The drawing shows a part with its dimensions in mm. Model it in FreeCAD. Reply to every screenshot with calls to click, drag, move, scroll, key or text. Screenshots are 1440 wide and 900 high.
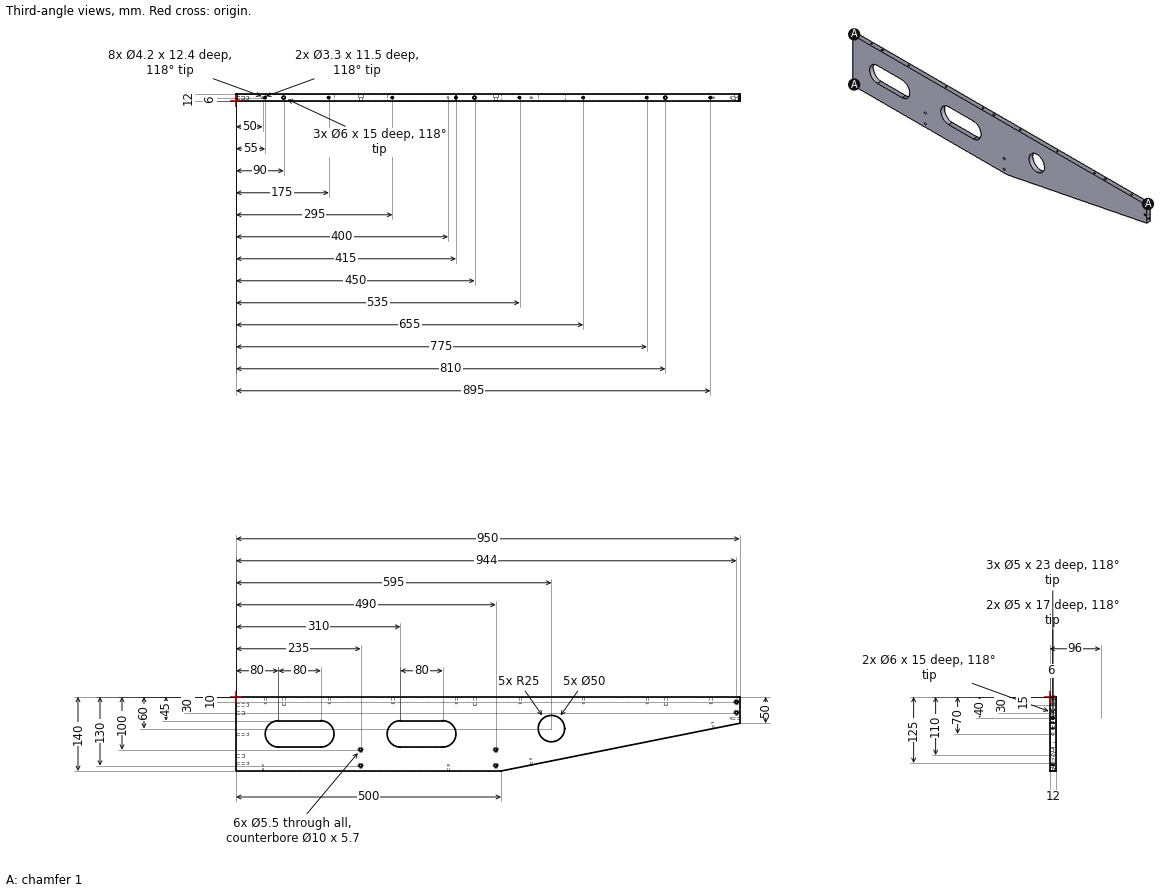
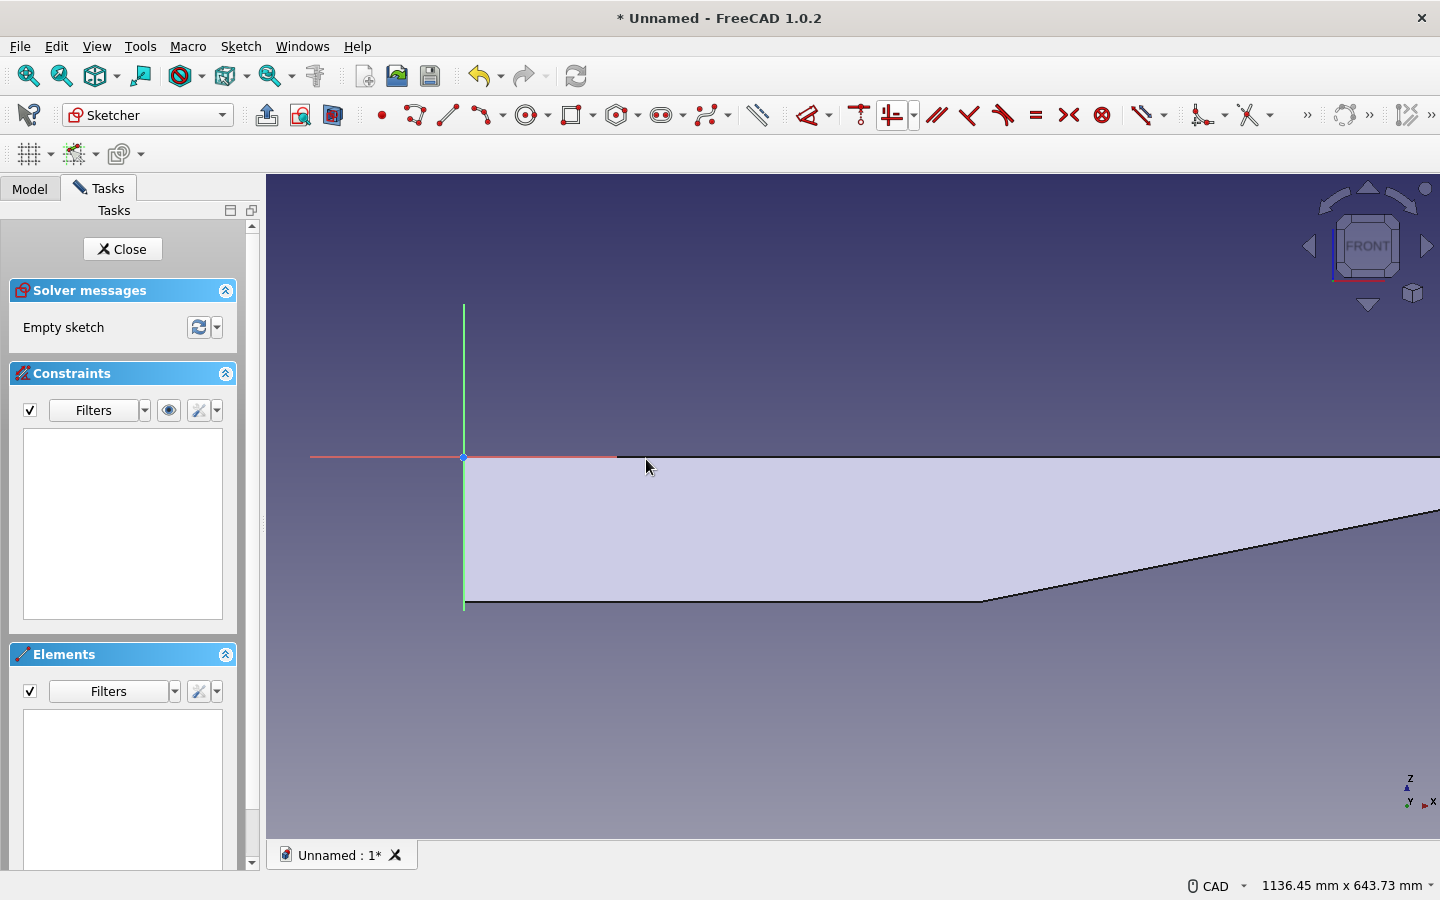
click(660, 116)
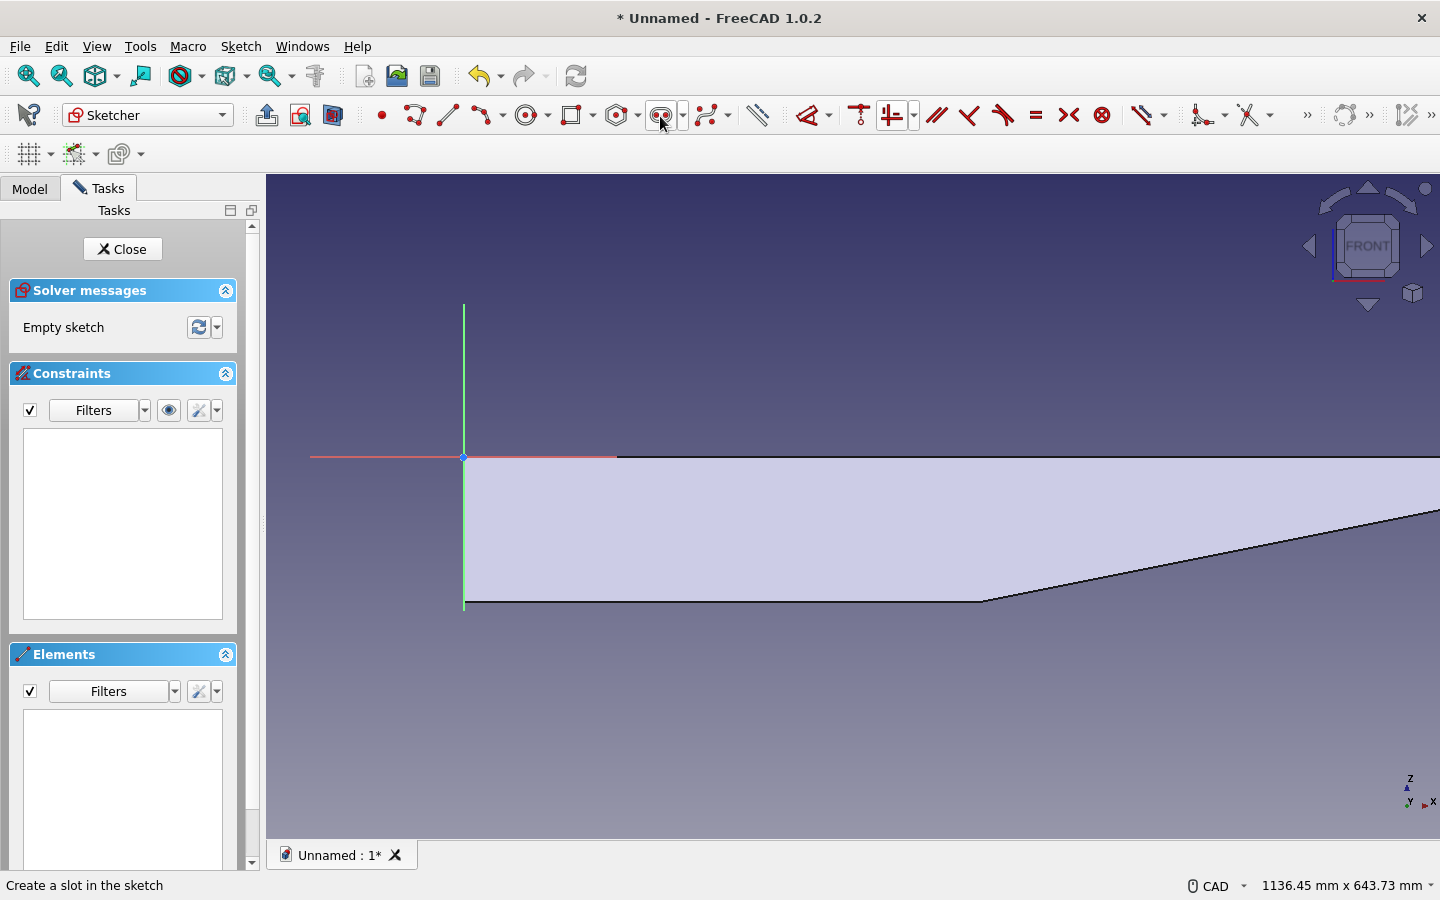
click(547, 530)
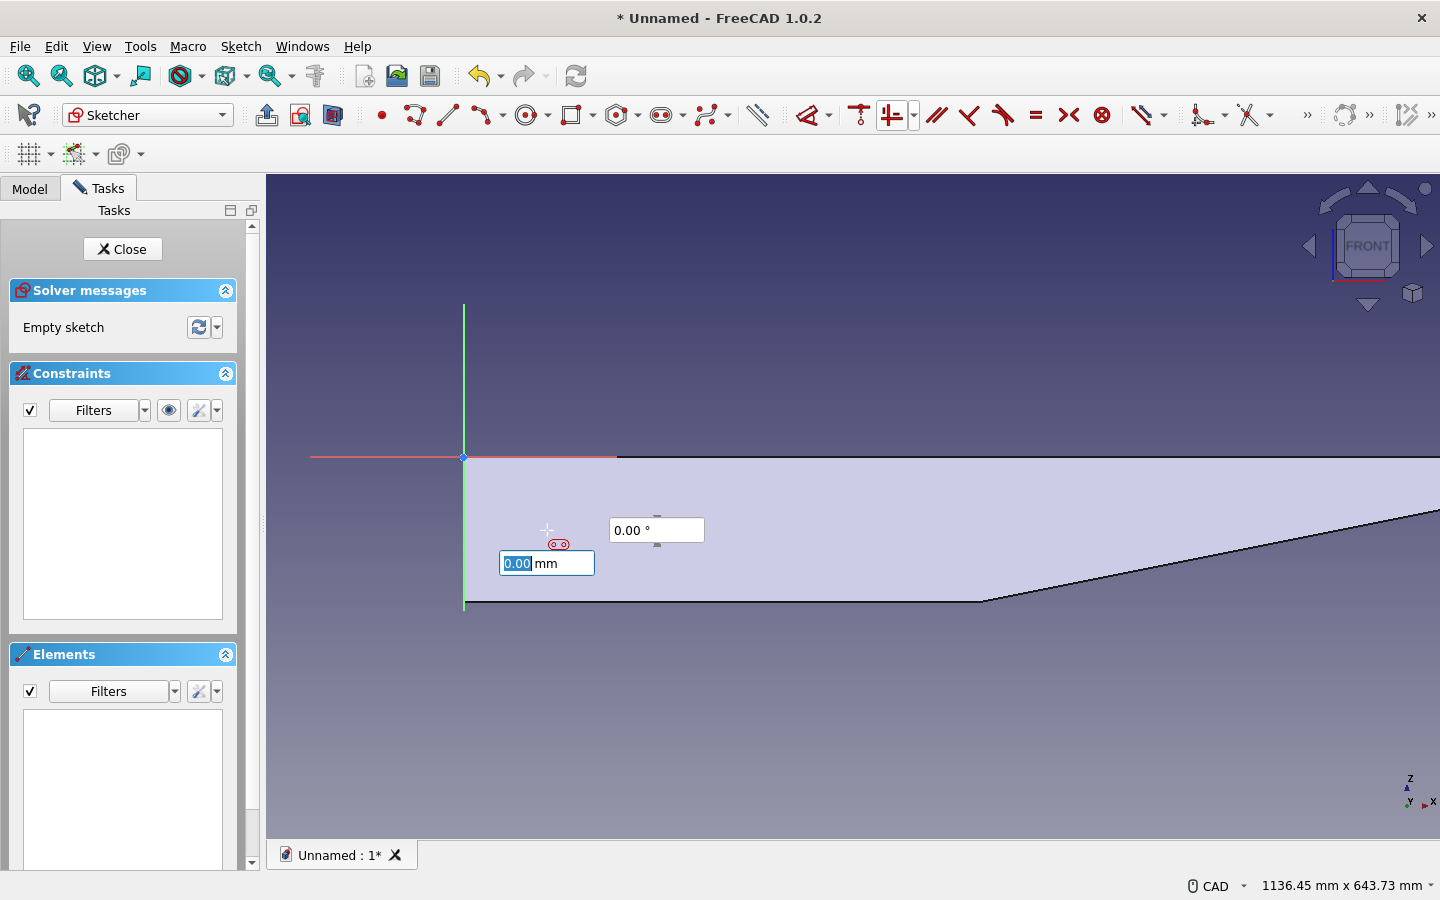
click(629, 530)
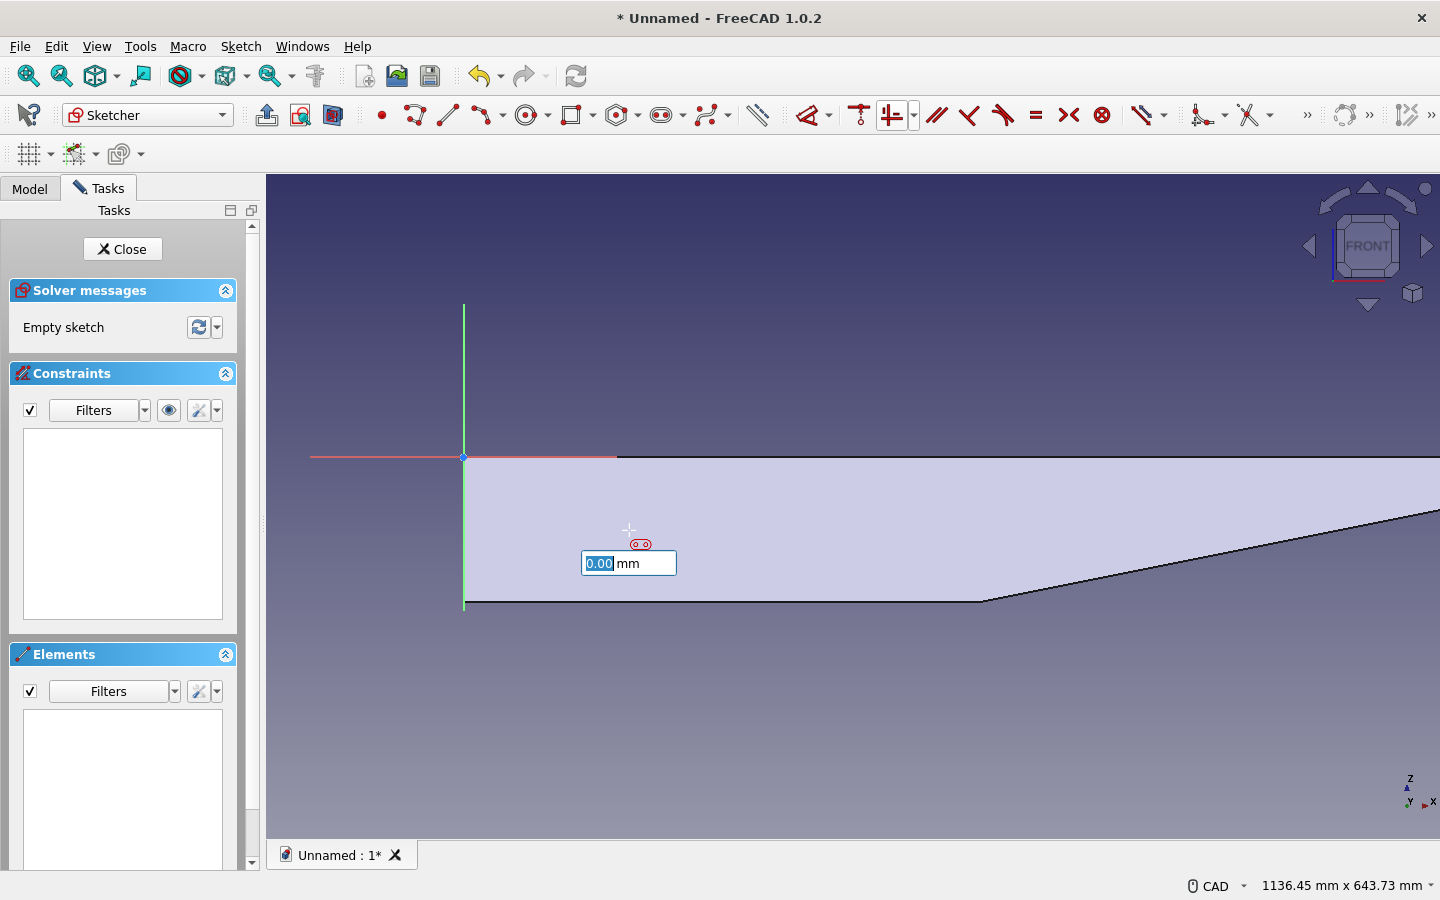
click(588, 504)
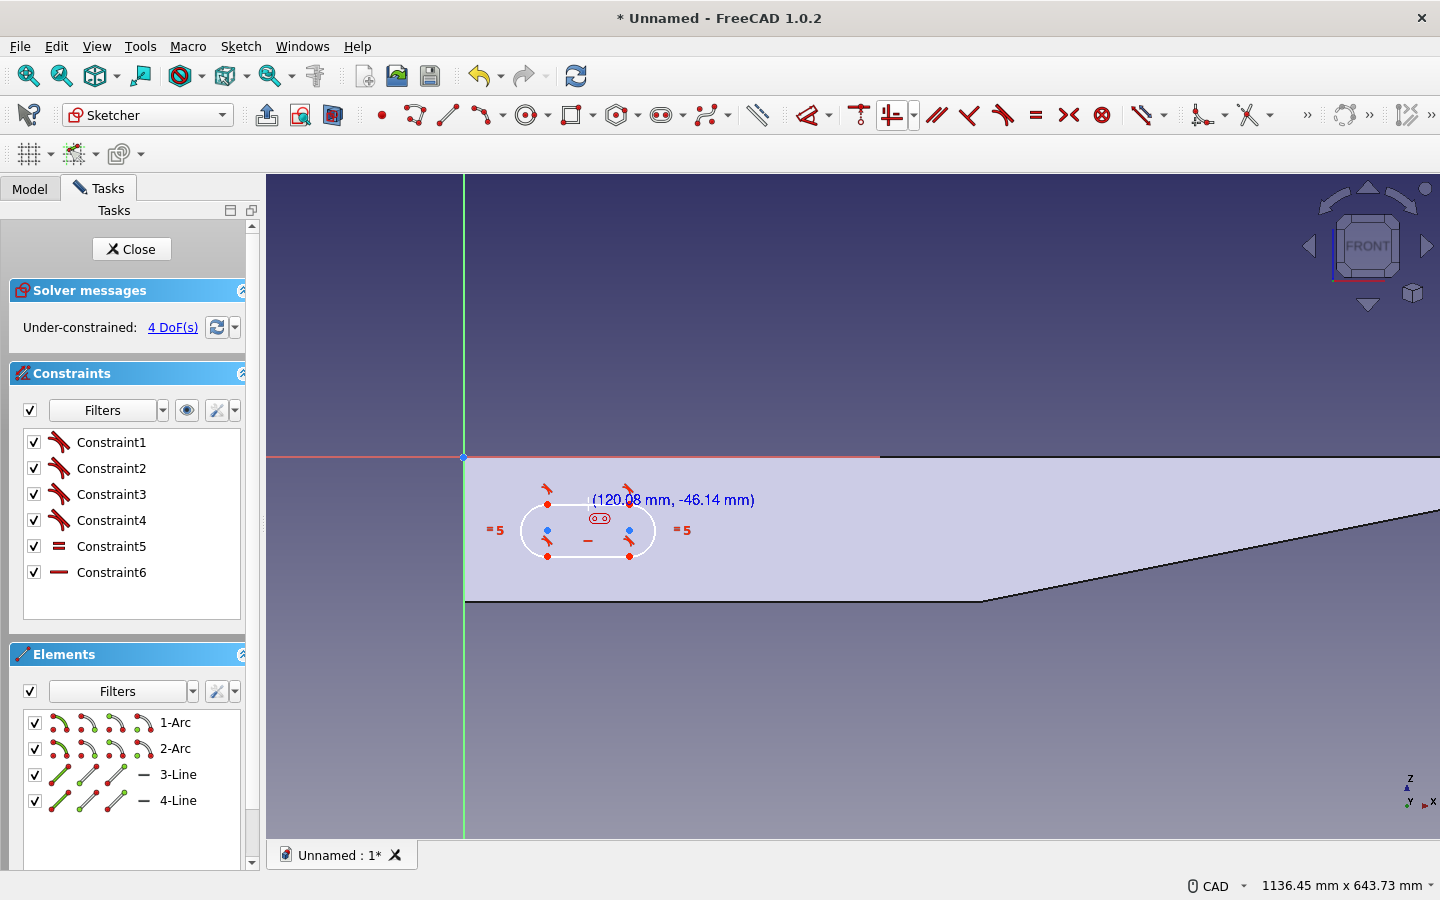
click(784, 530)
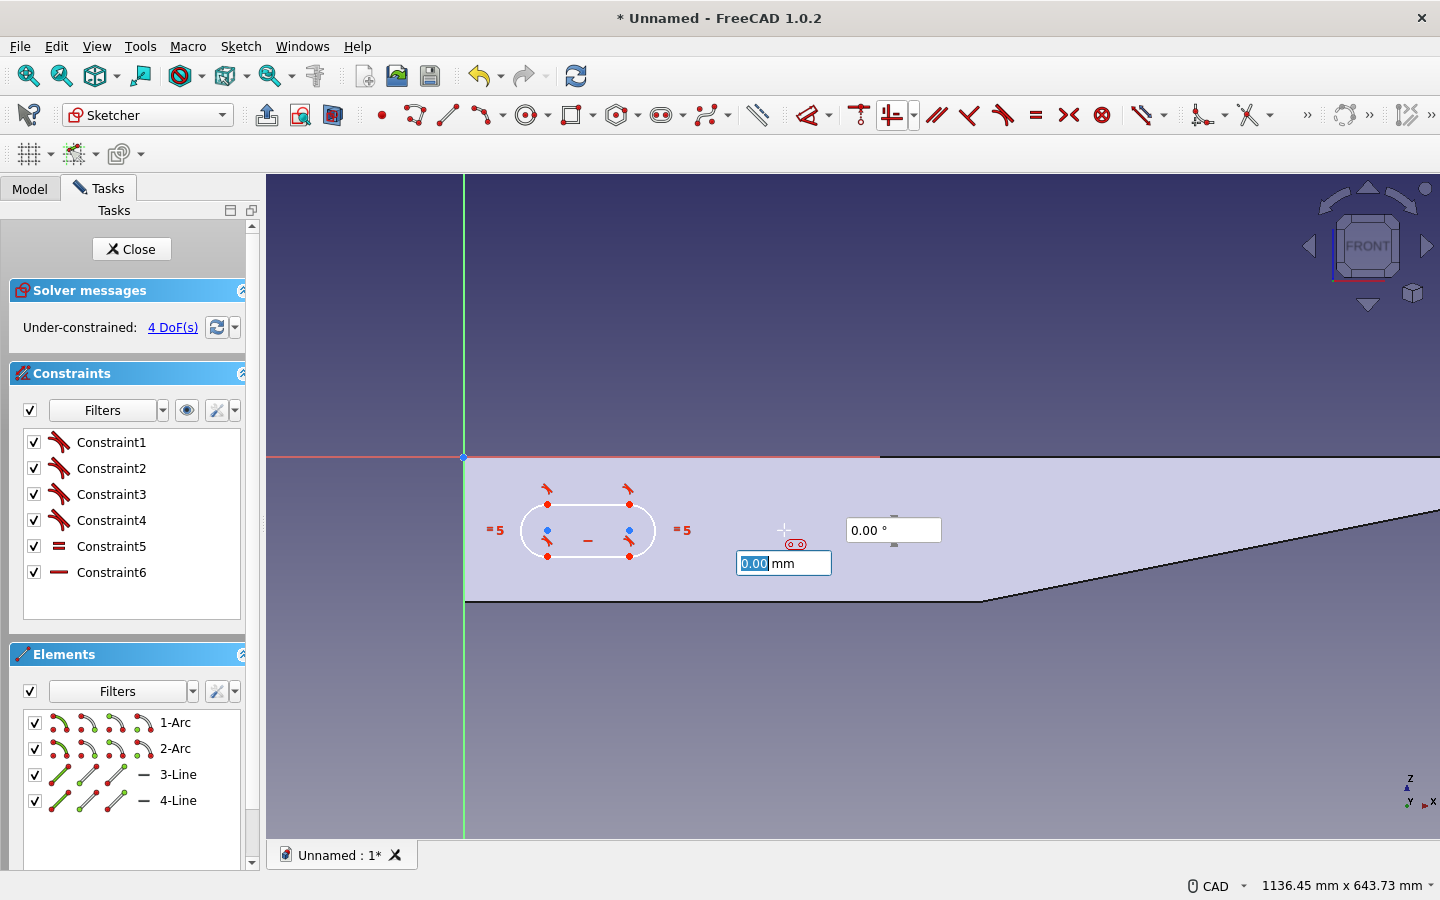
click(867, 530)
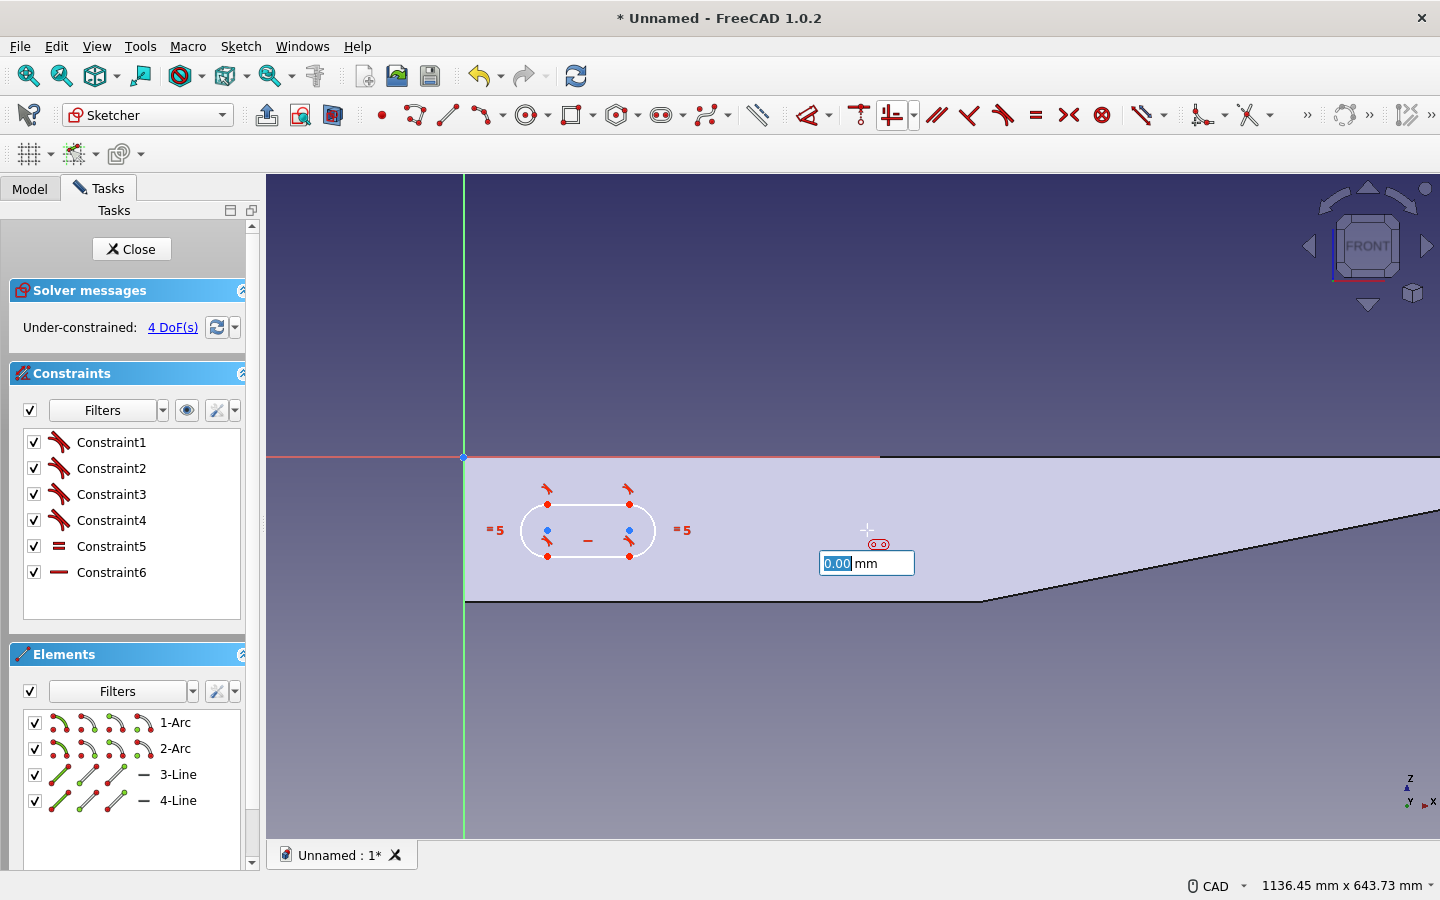
click(826, 504)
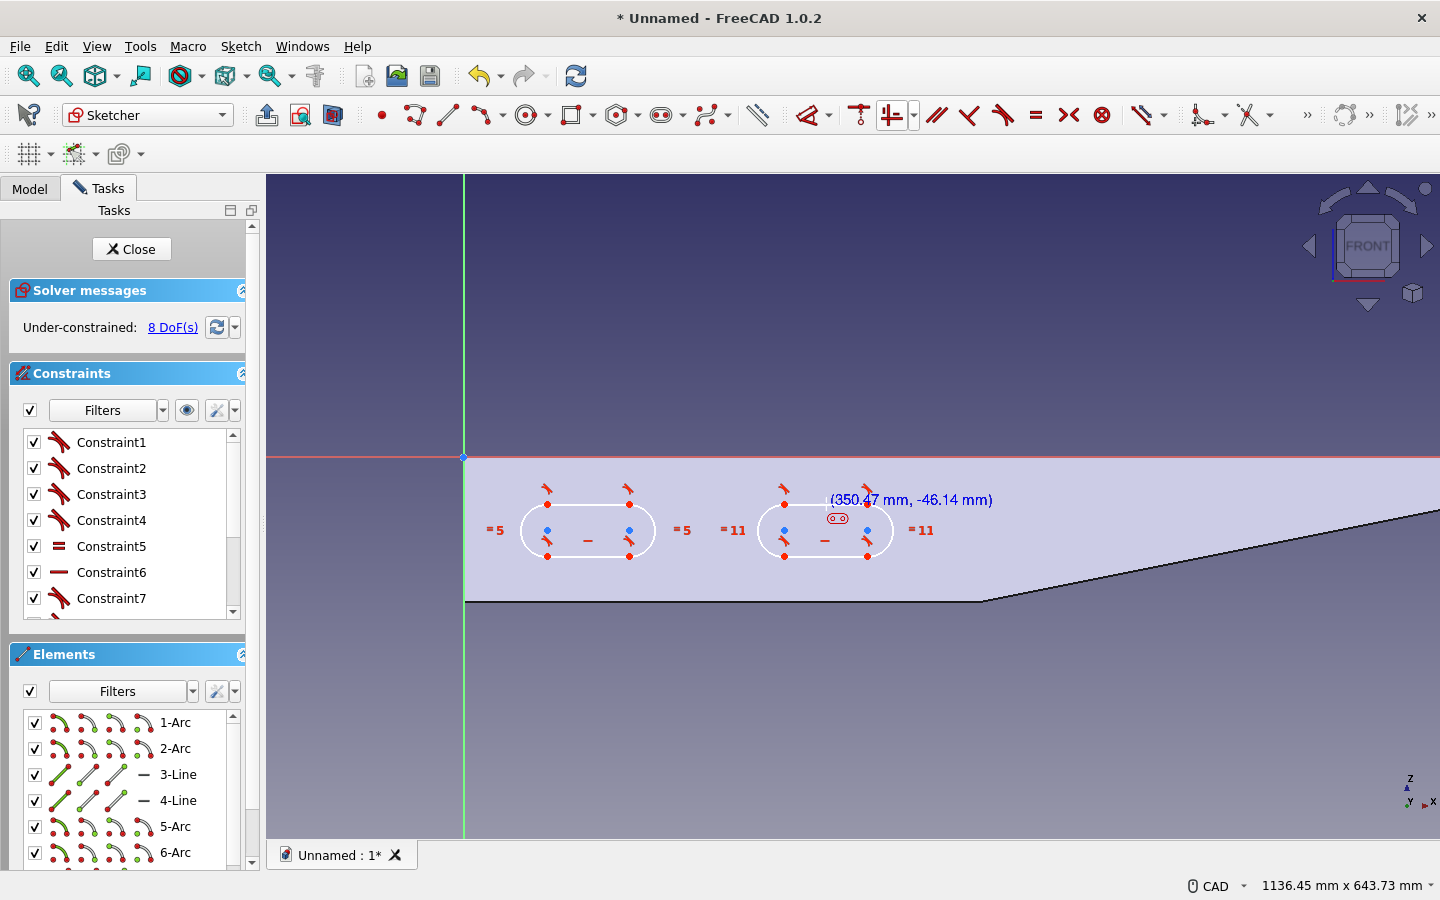
click(526, 116)